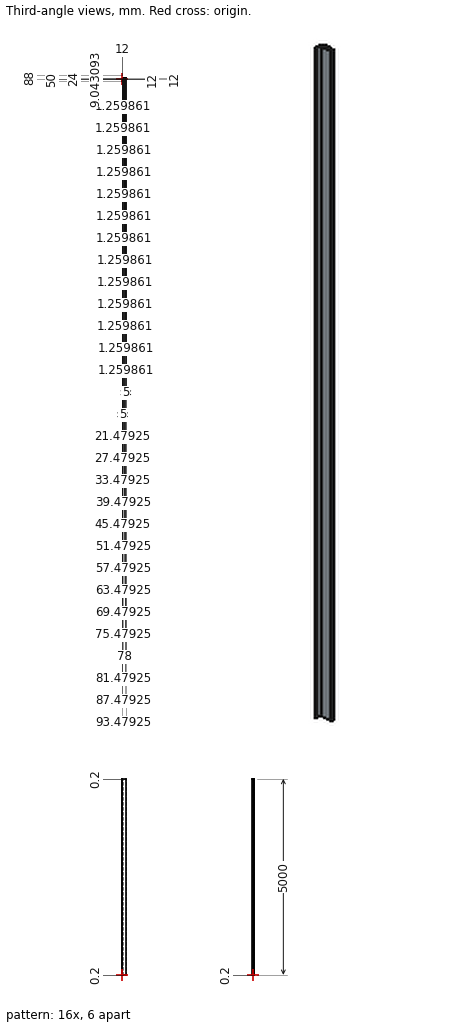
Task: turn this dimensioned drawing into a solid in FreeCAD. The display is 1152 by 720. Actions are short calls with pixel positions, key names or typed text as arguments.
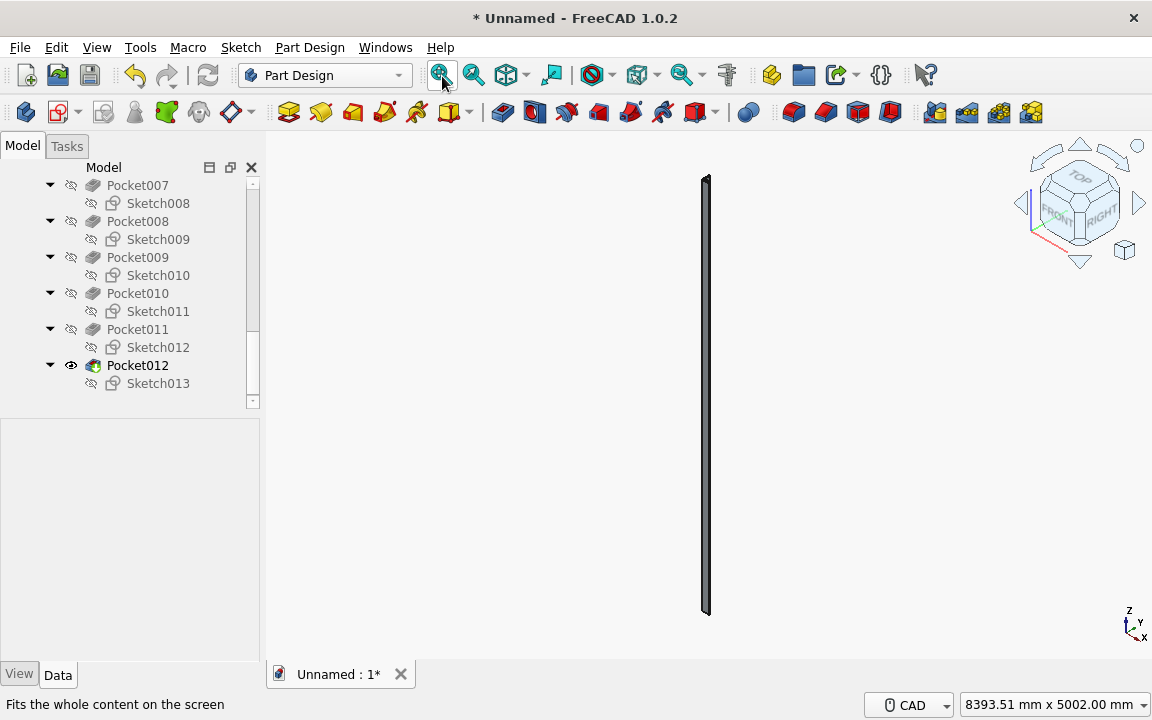
scroll(708, 182, up, 14)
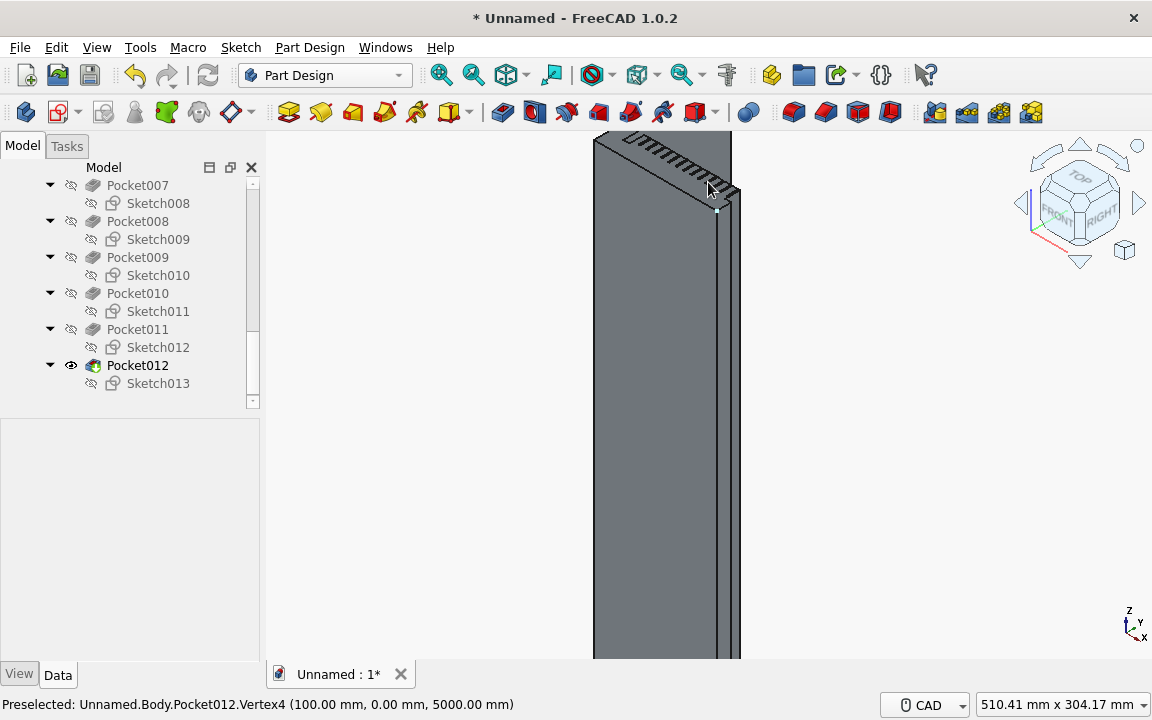
click(682, 179)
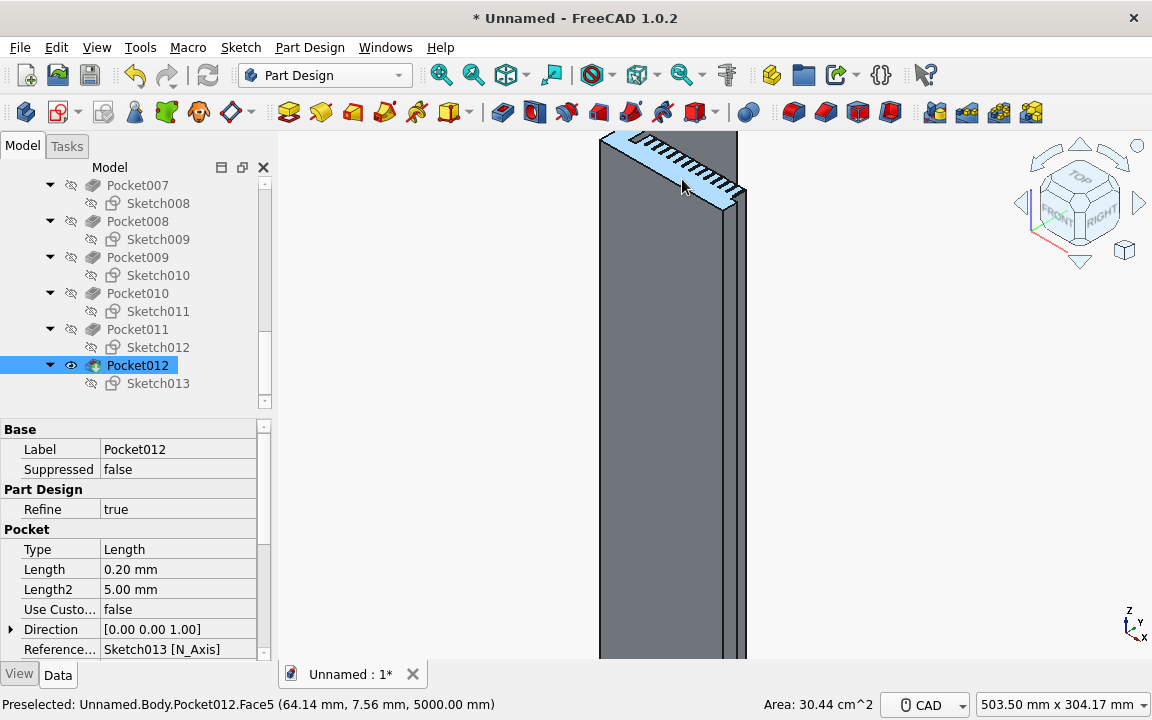
click(58, 112)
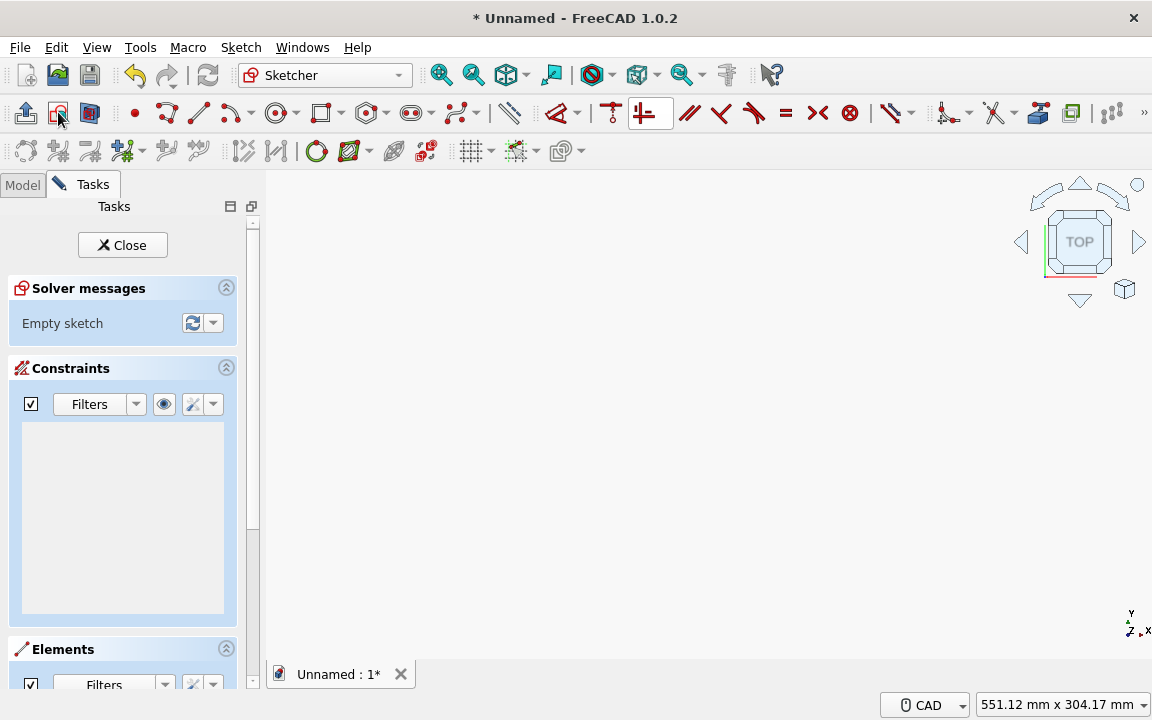
scroll(640, 414, down, 5)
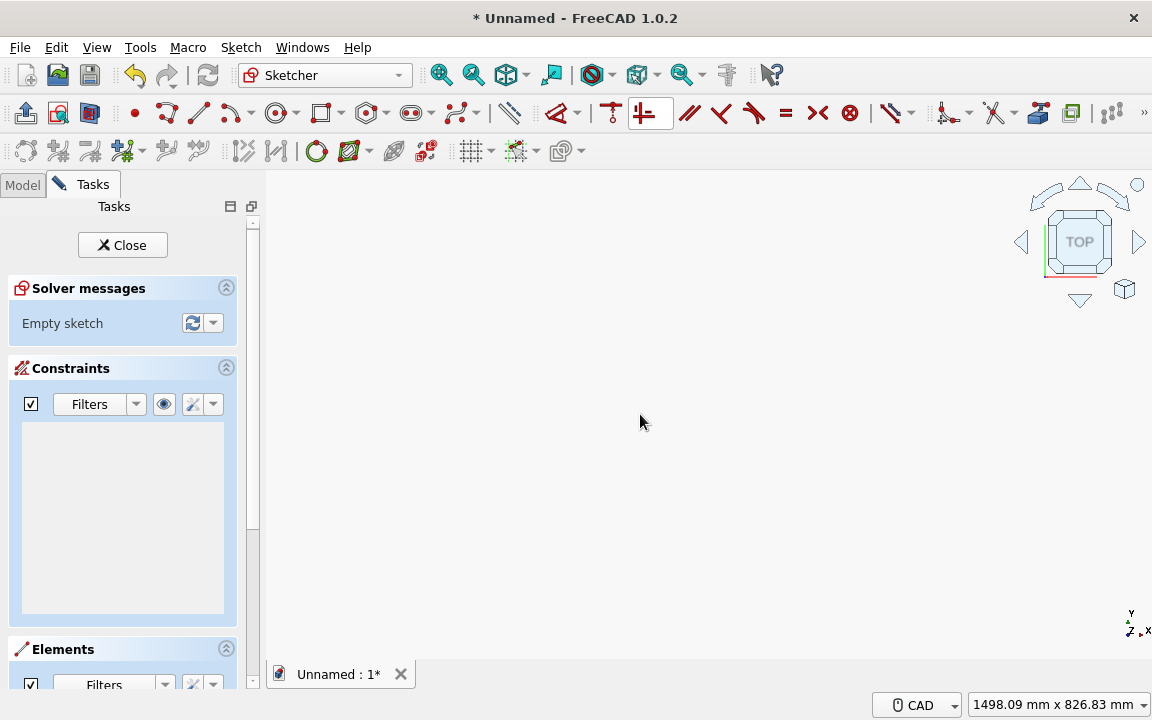
scroll(640, 414, down, 5)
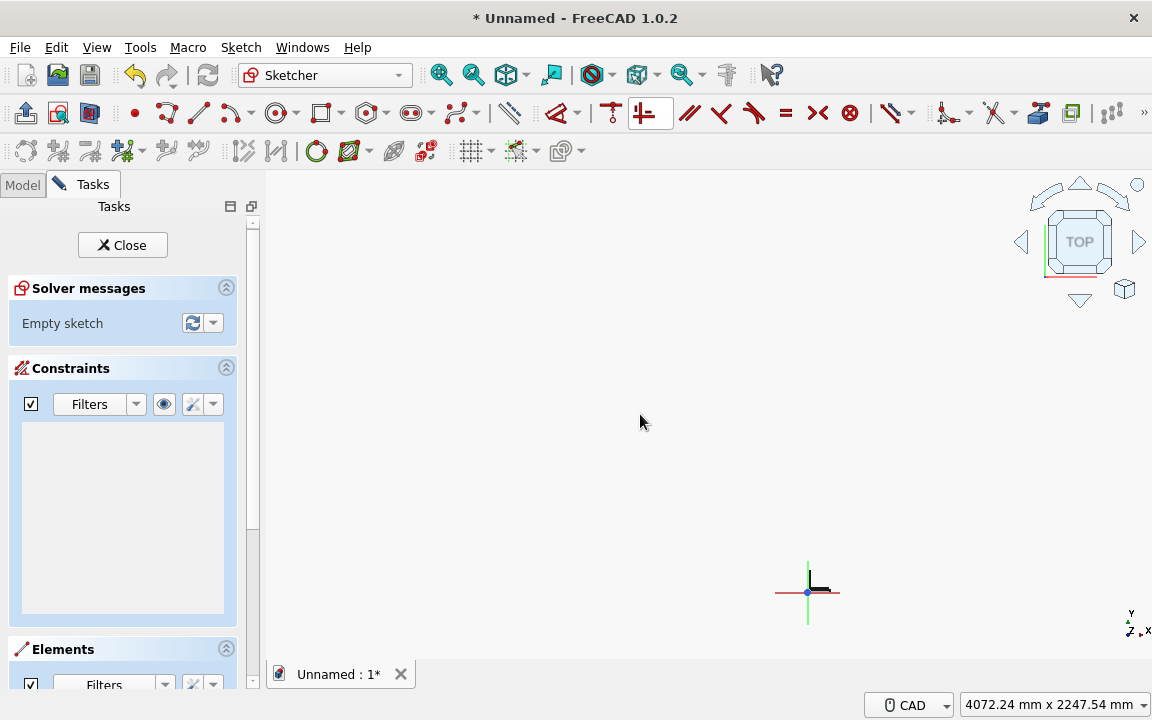
scroll(818, 605, up, 15)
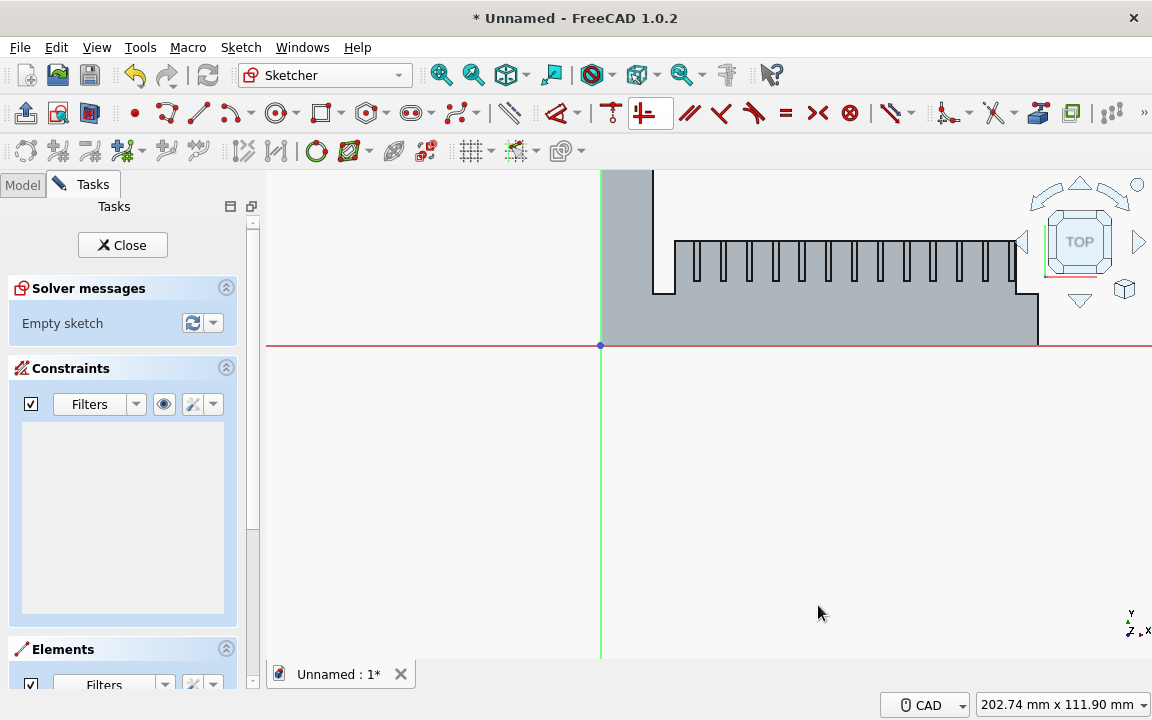
scroll(599, 379, up, 2)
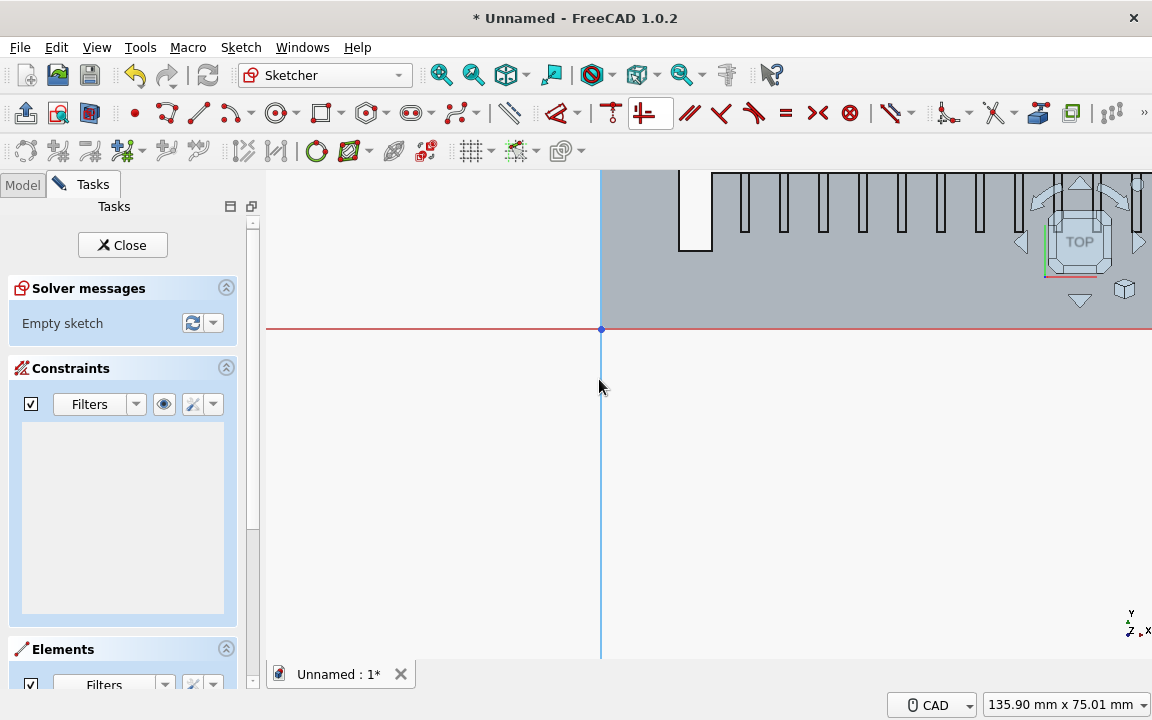
click(322, 114)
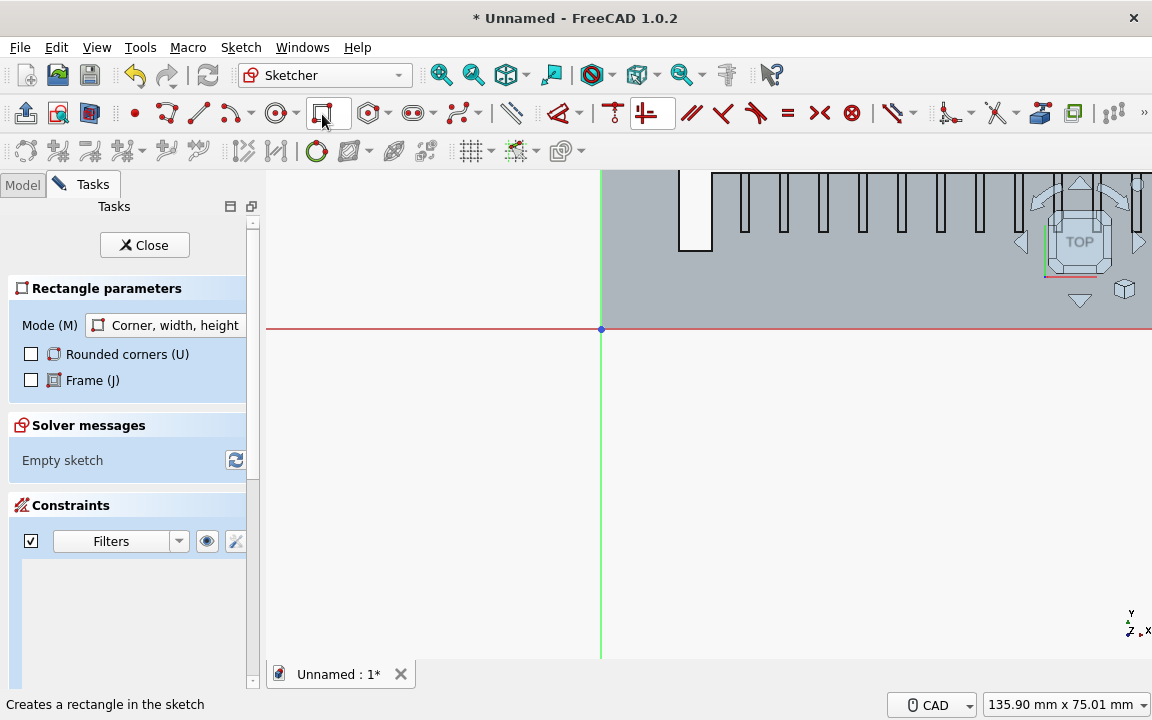
click(601, 251)
click(679, 577)
key(Escape)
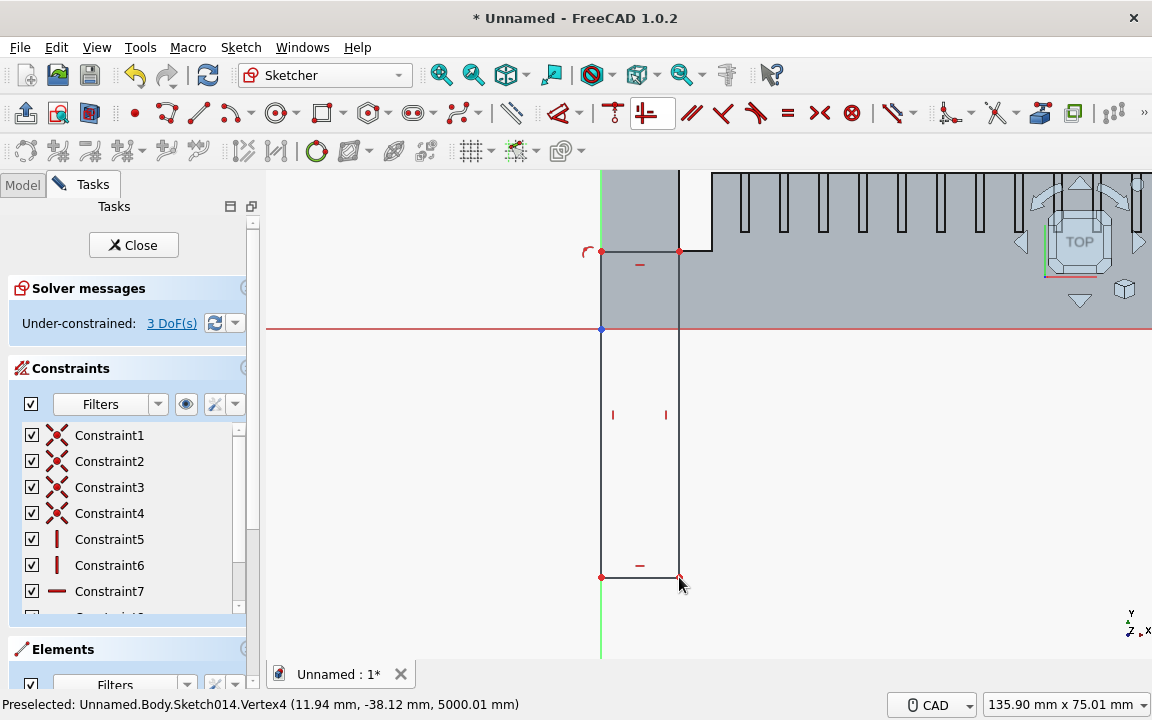
click(558, 114)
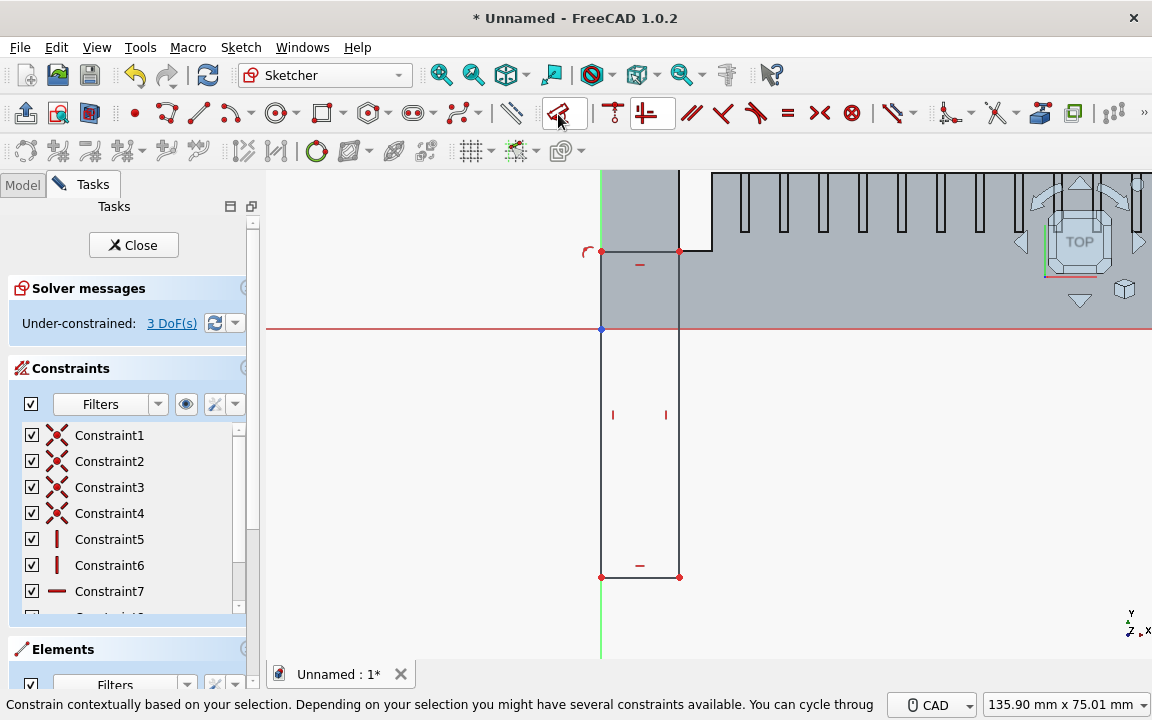
click(601, 350)
click(567, 415)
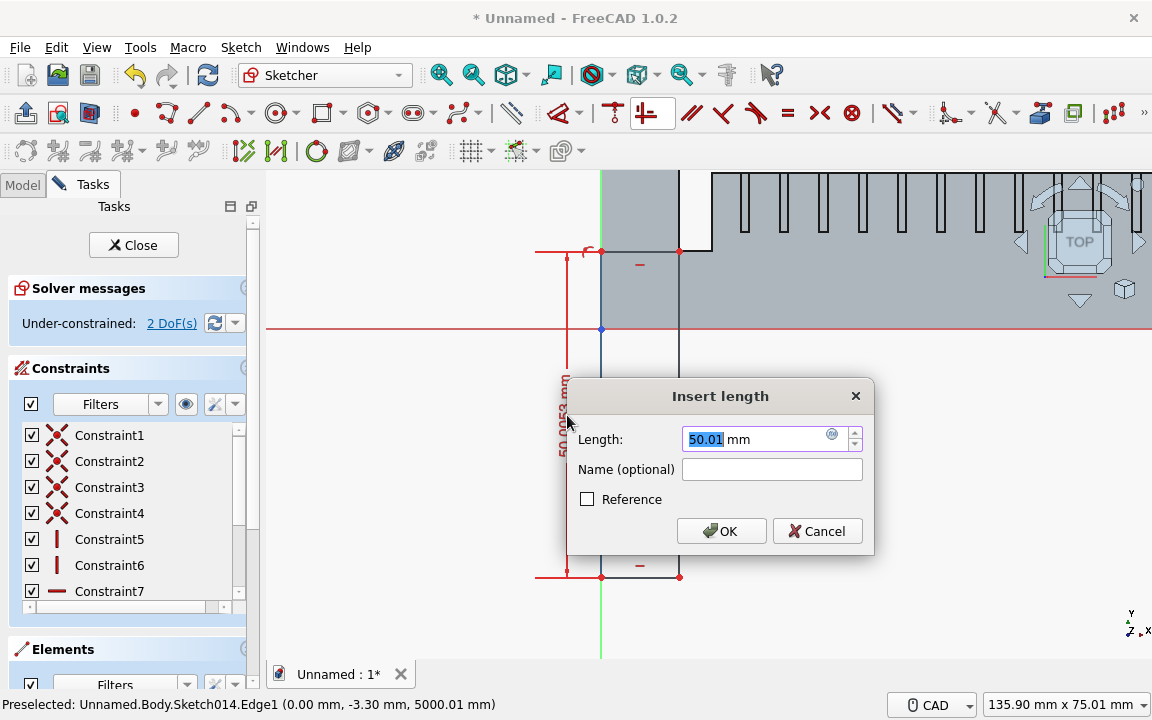
text(50)
key(Return)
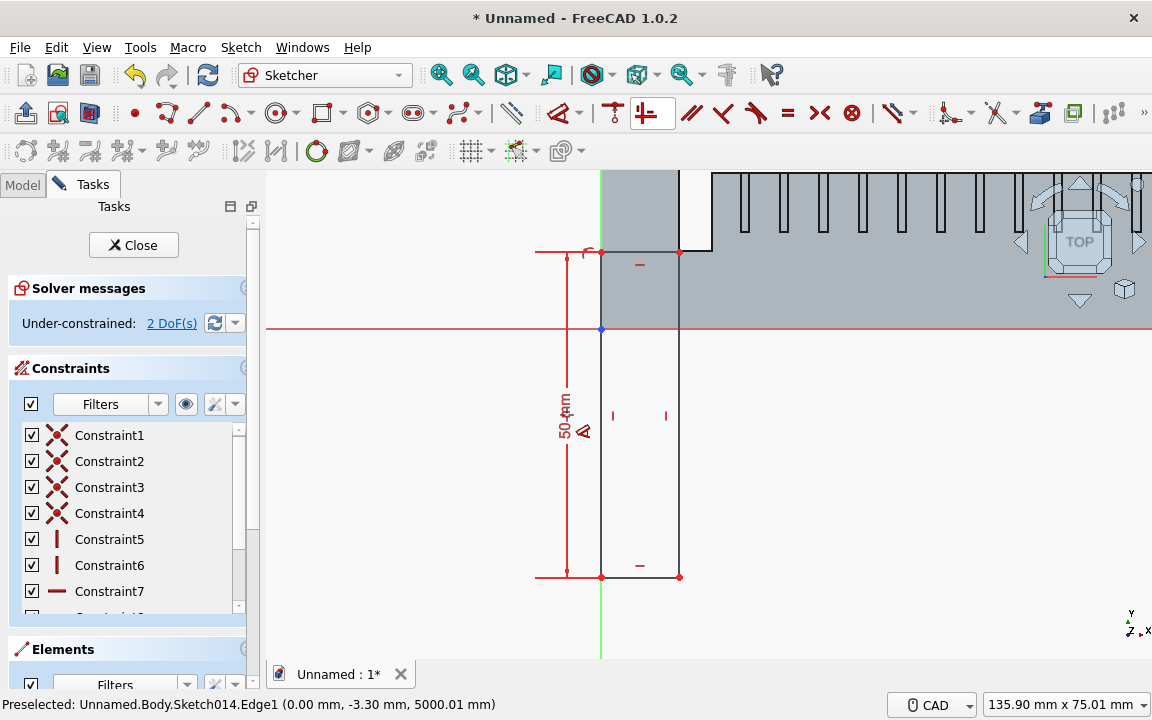
click(624, 578)
click(640, 612)